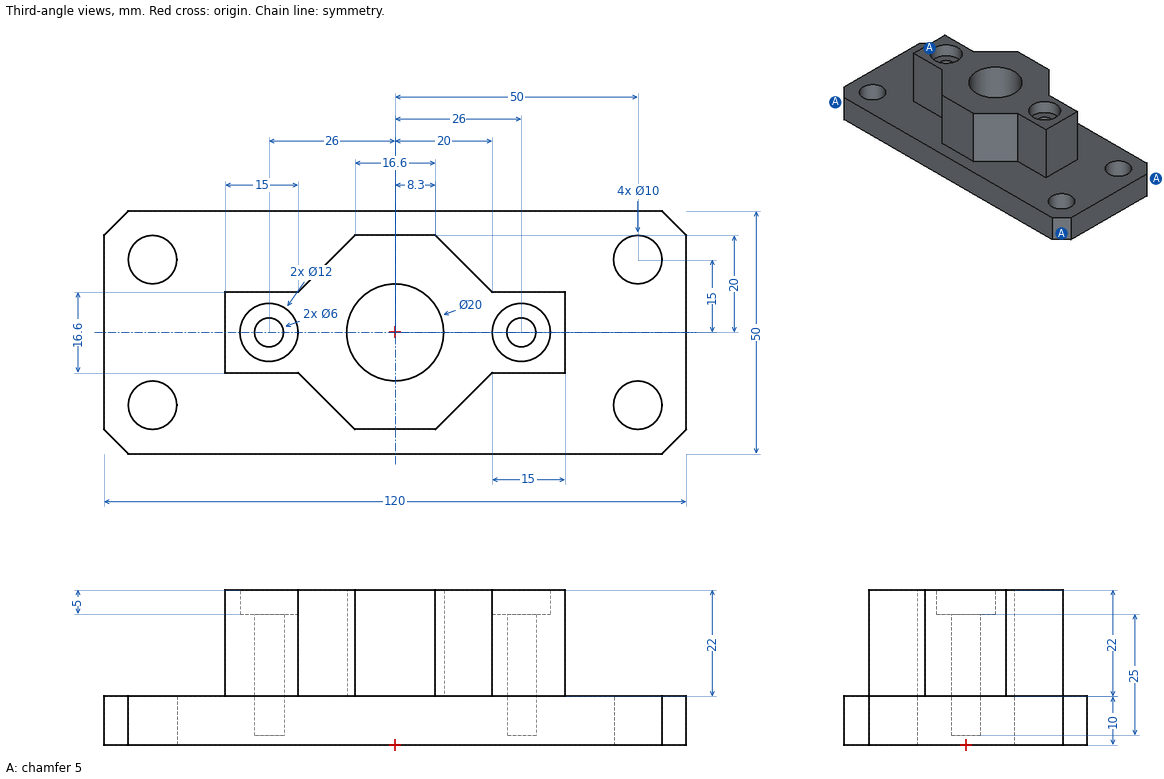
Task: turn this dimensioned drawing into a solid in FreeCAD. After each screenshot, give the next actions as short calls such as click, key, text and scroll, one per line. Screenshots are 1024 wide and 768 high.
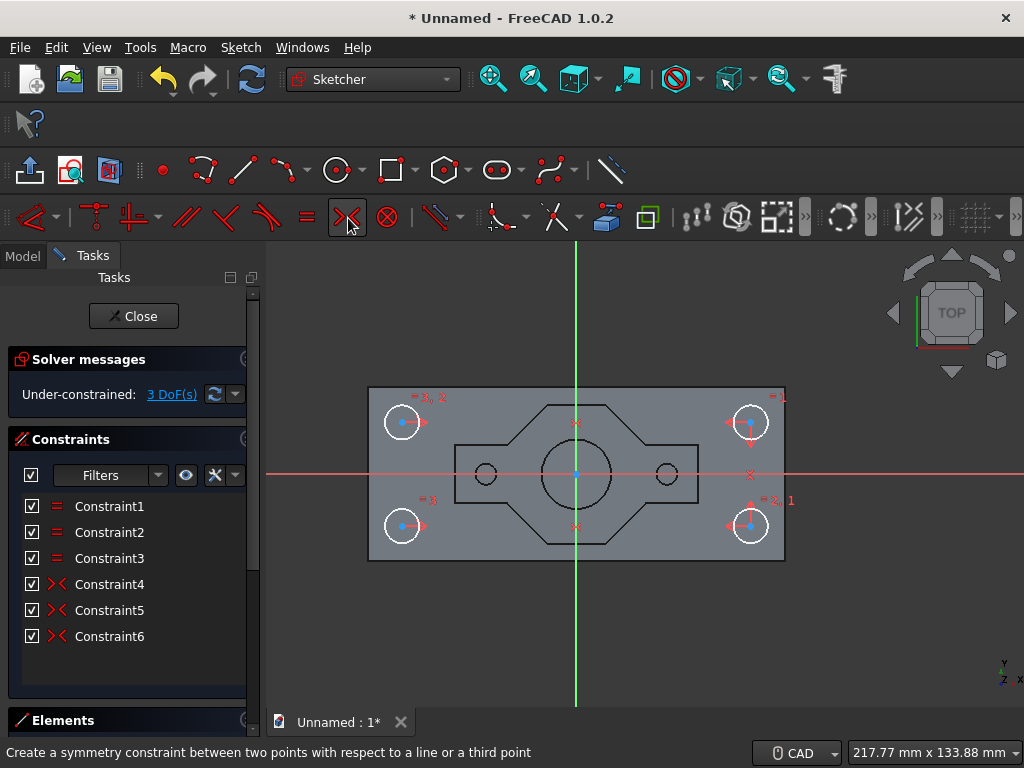
click(32, 218)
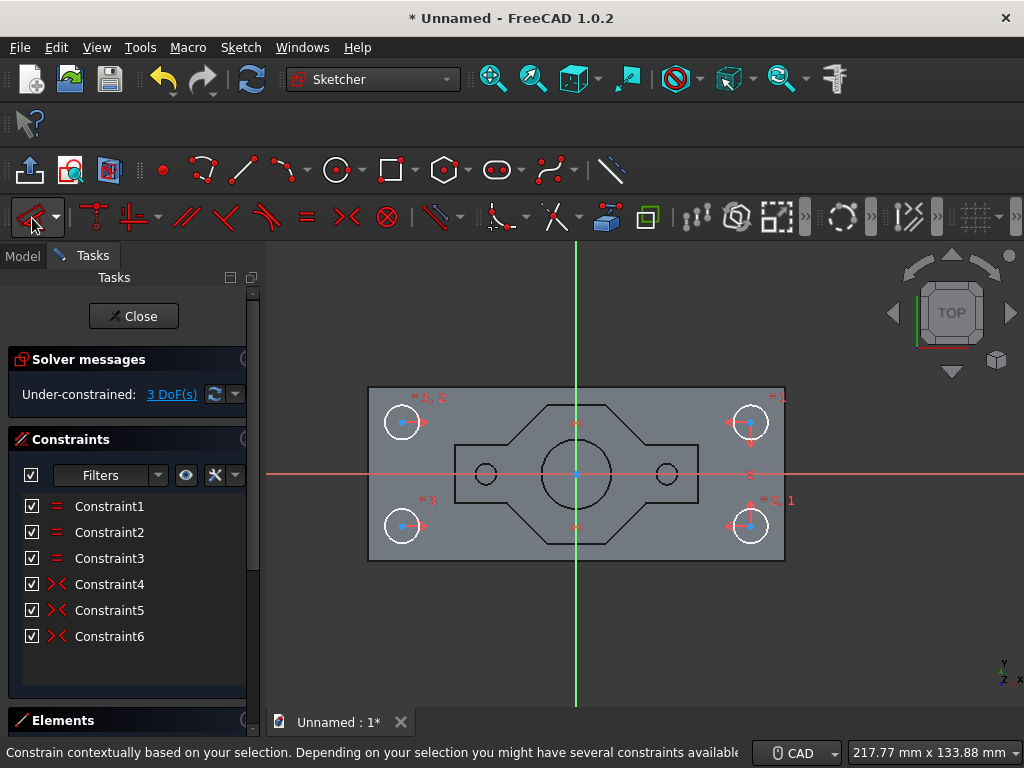
click(763, 410)
click(785, 387)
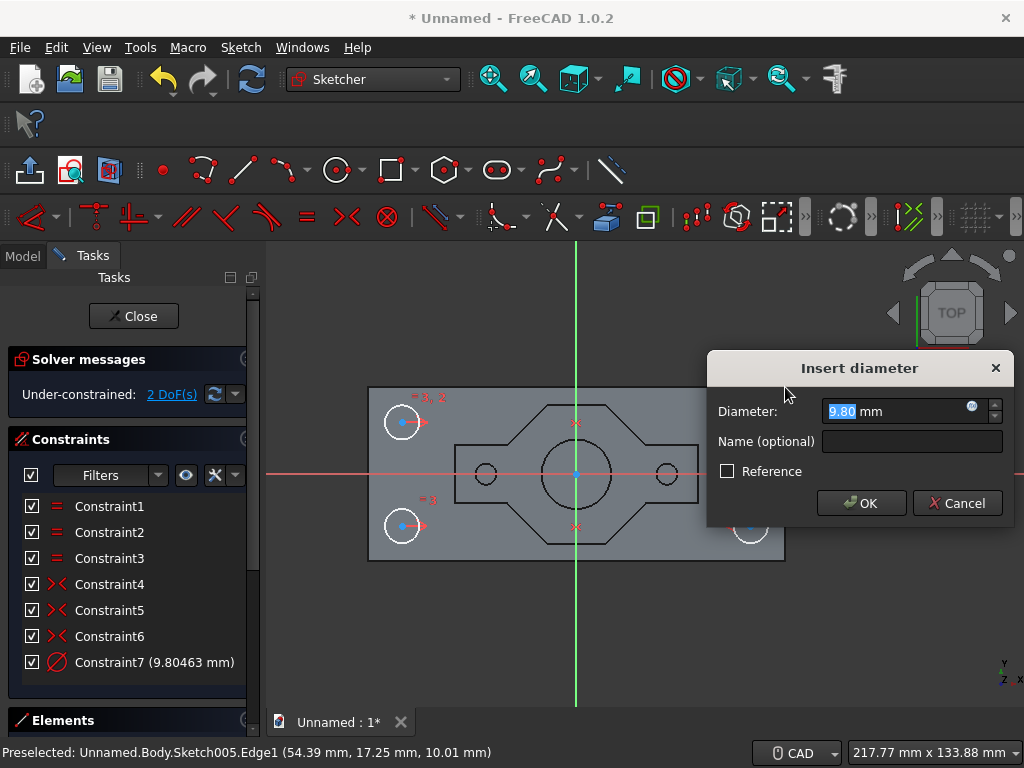
text(10)
key(Return)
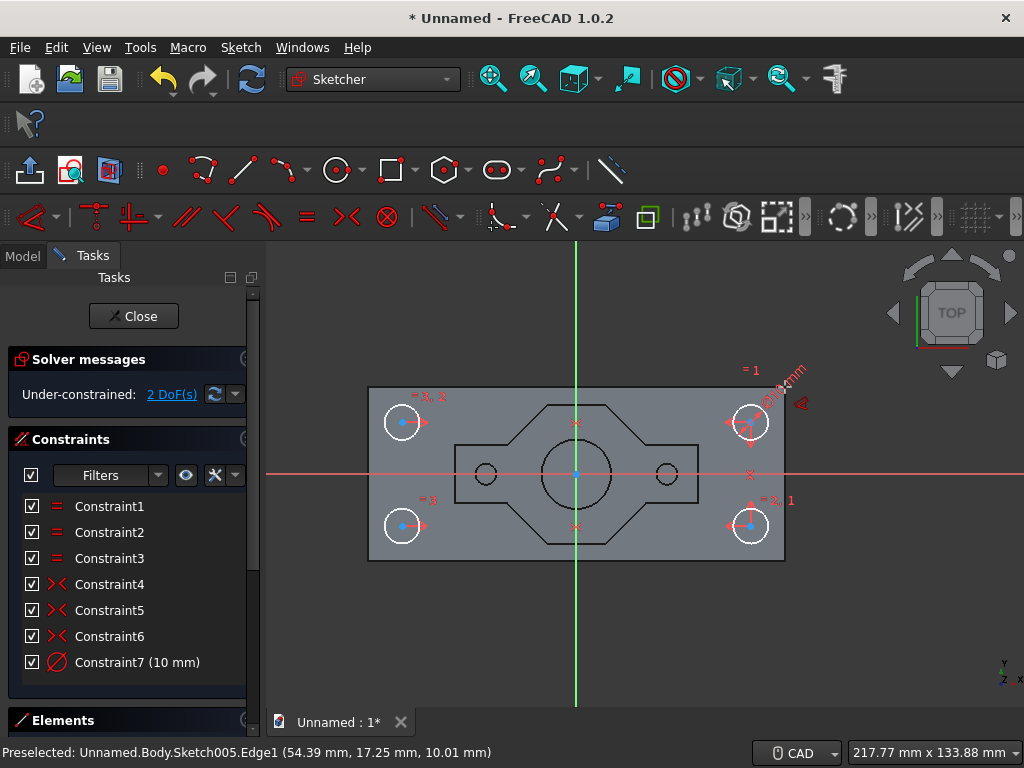
click(751, 422)
click(664, 388)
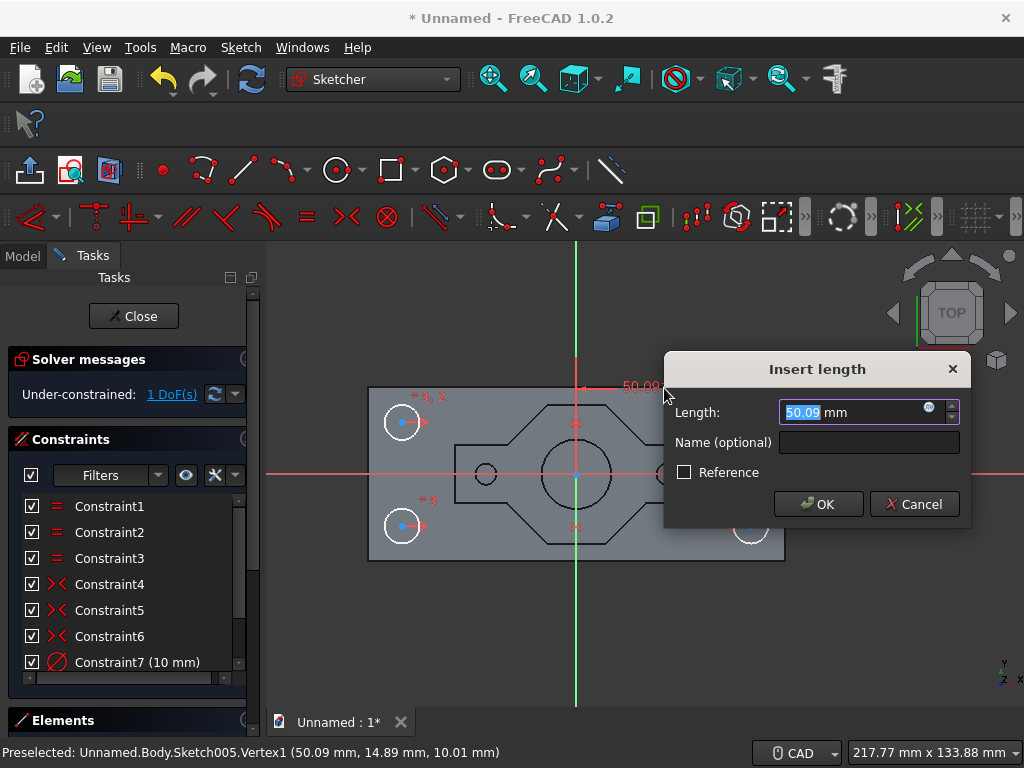
text(50)
key(Return)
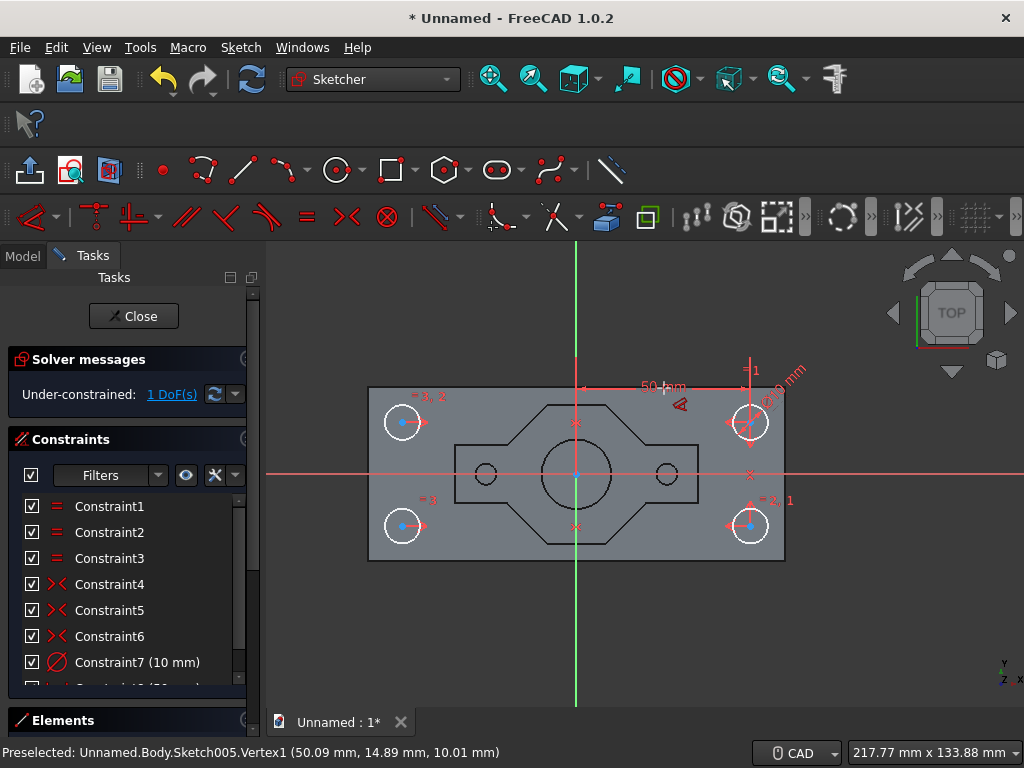
click(750, 422)
click(784, 448)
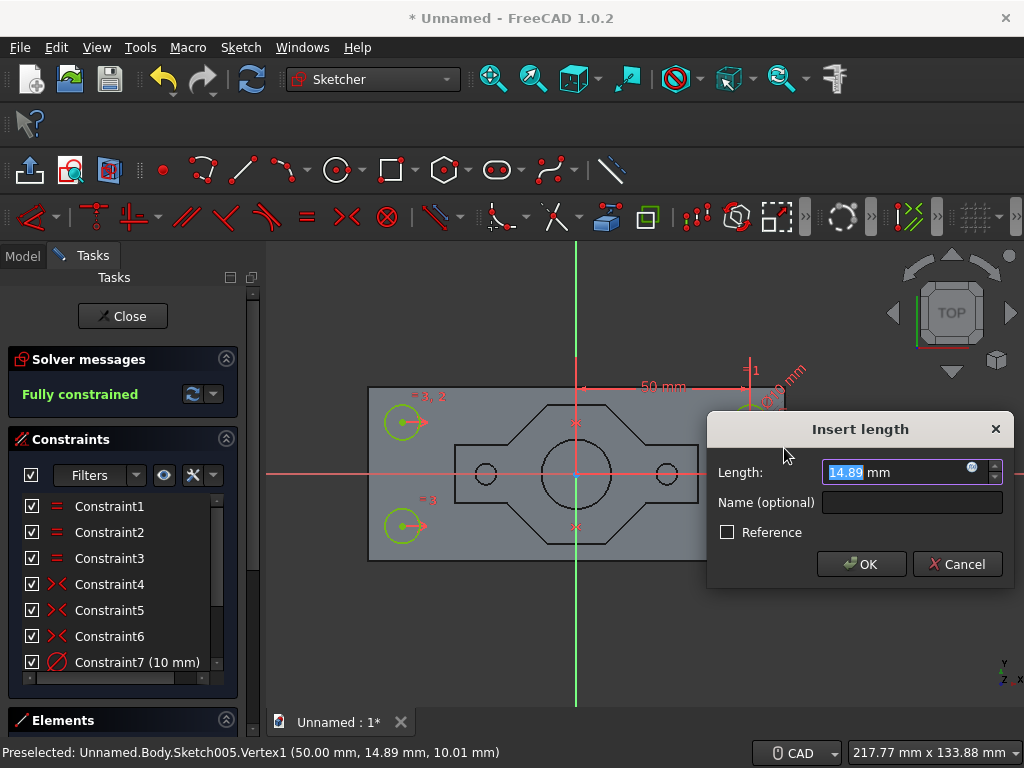
text(15)
key(Return)
key(Escape)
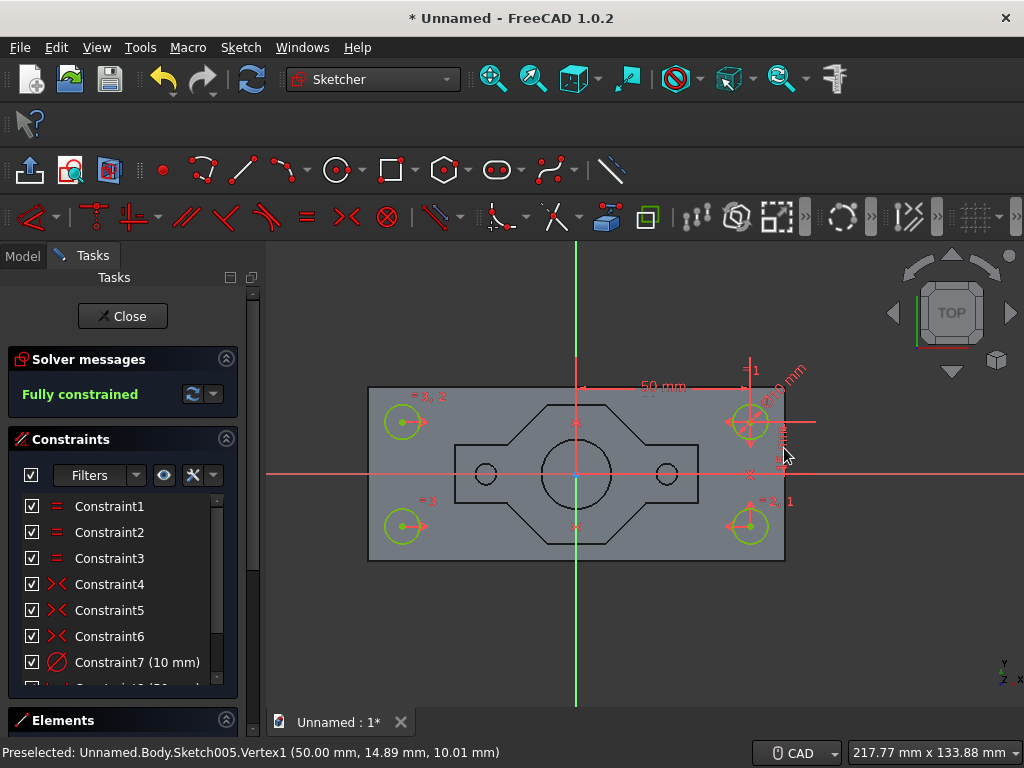
click(123, 316)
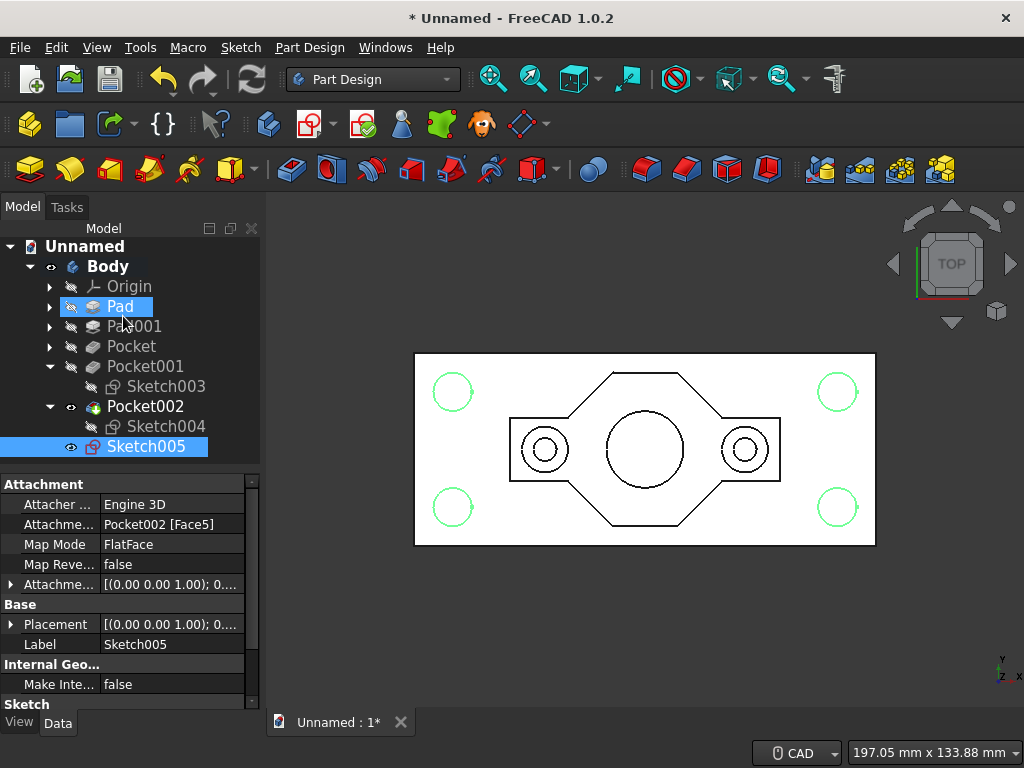
click(292, 170)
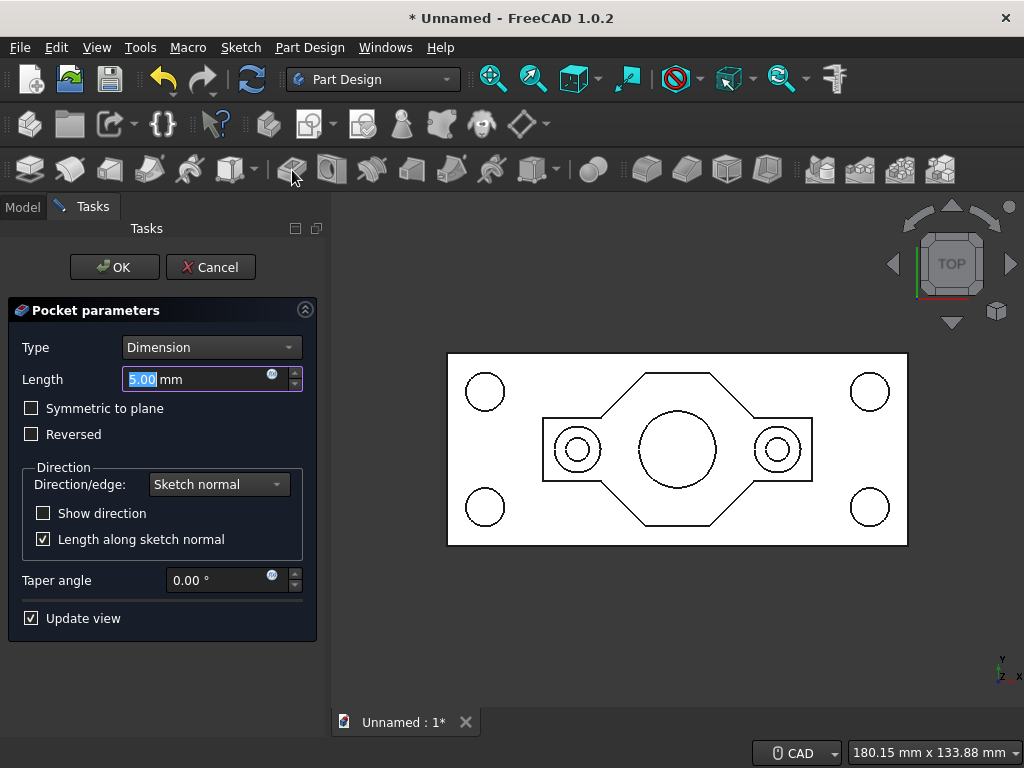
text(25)
key(Tab)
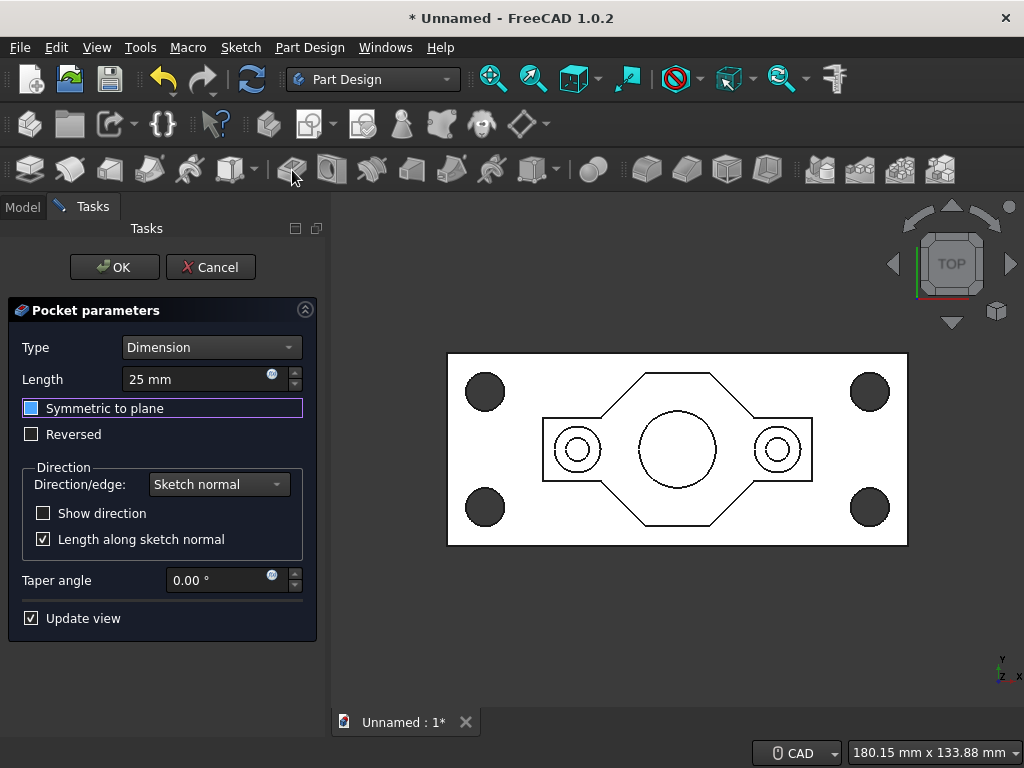
click(115, 267)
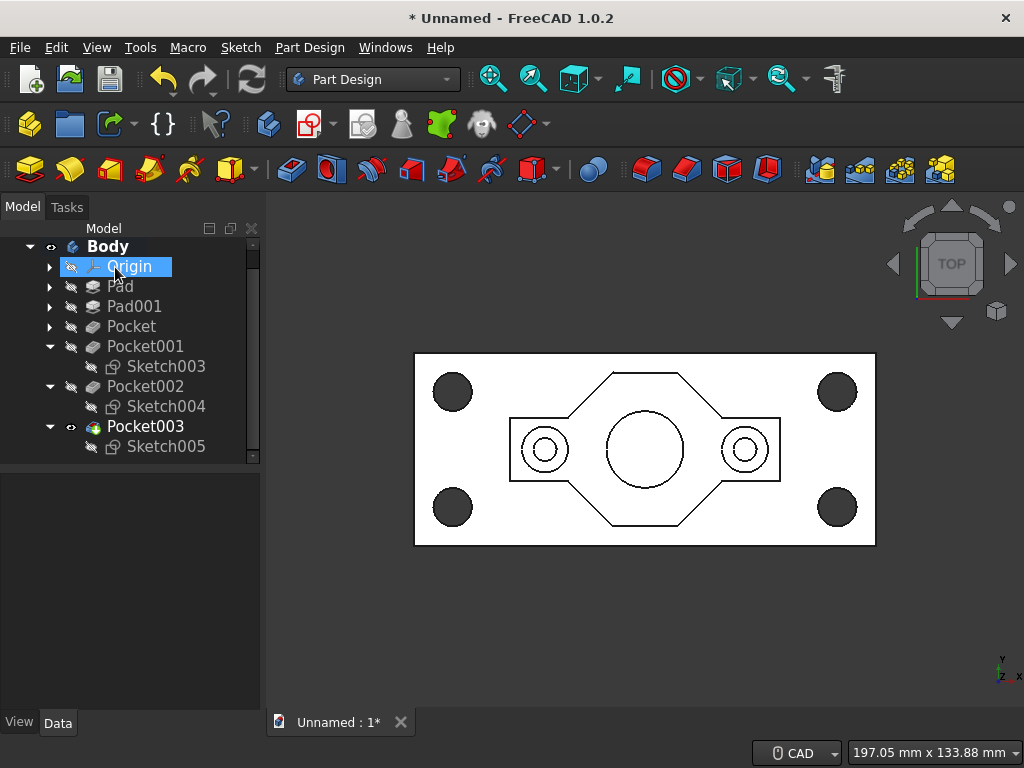
key(0)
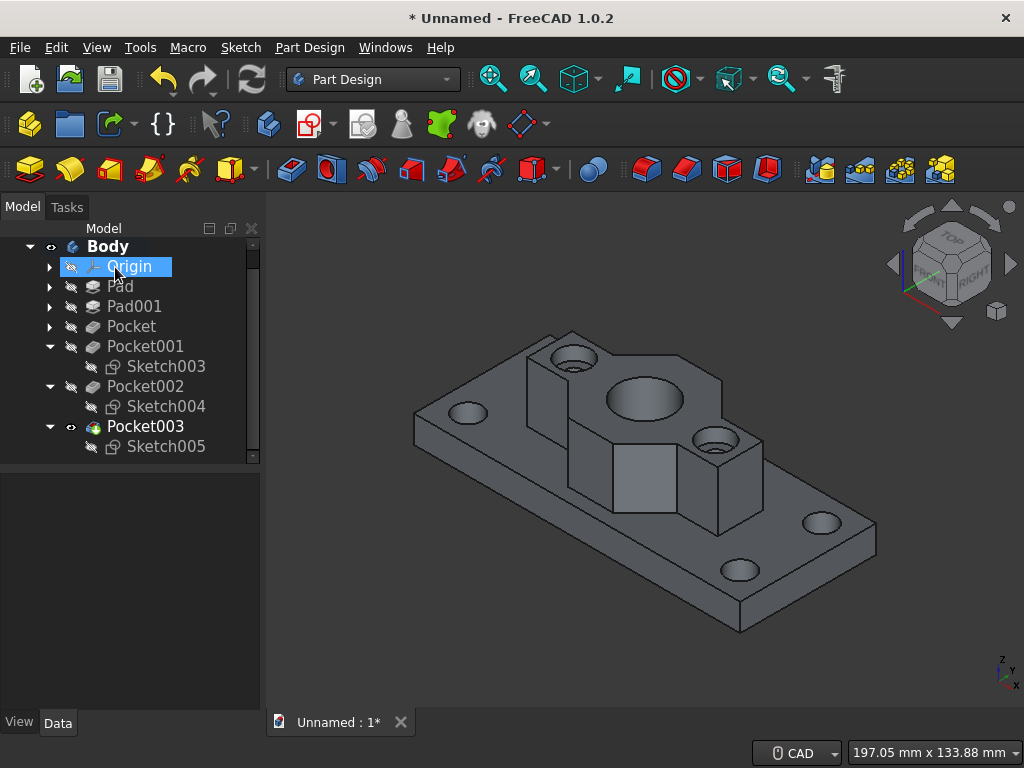
click(740, 617)